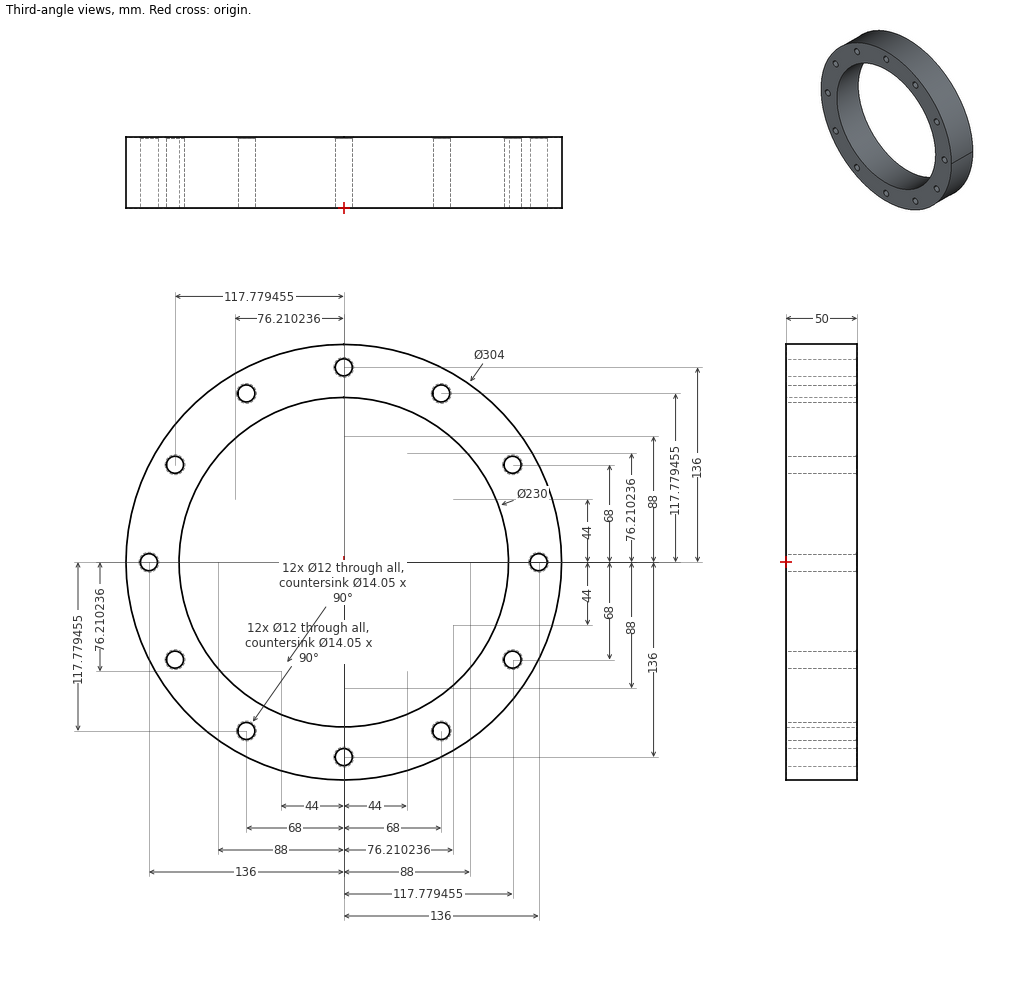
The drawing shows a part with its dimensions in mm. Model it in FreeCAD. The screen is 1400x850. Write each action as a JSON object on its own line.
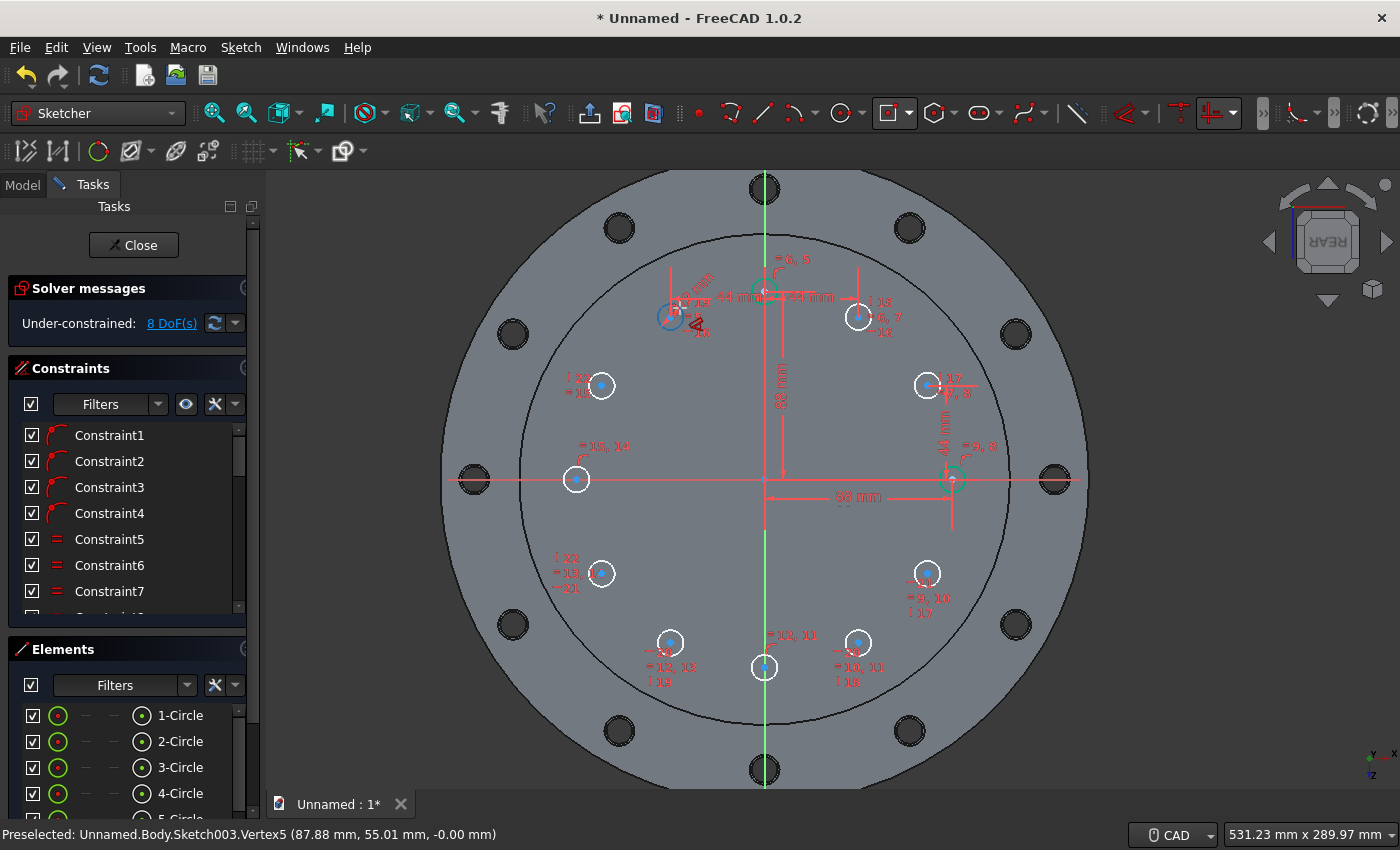
{"action": "left_click", "coordinate": [927, 574]}
{"action": "left_click", "coordinate": [961, 527]}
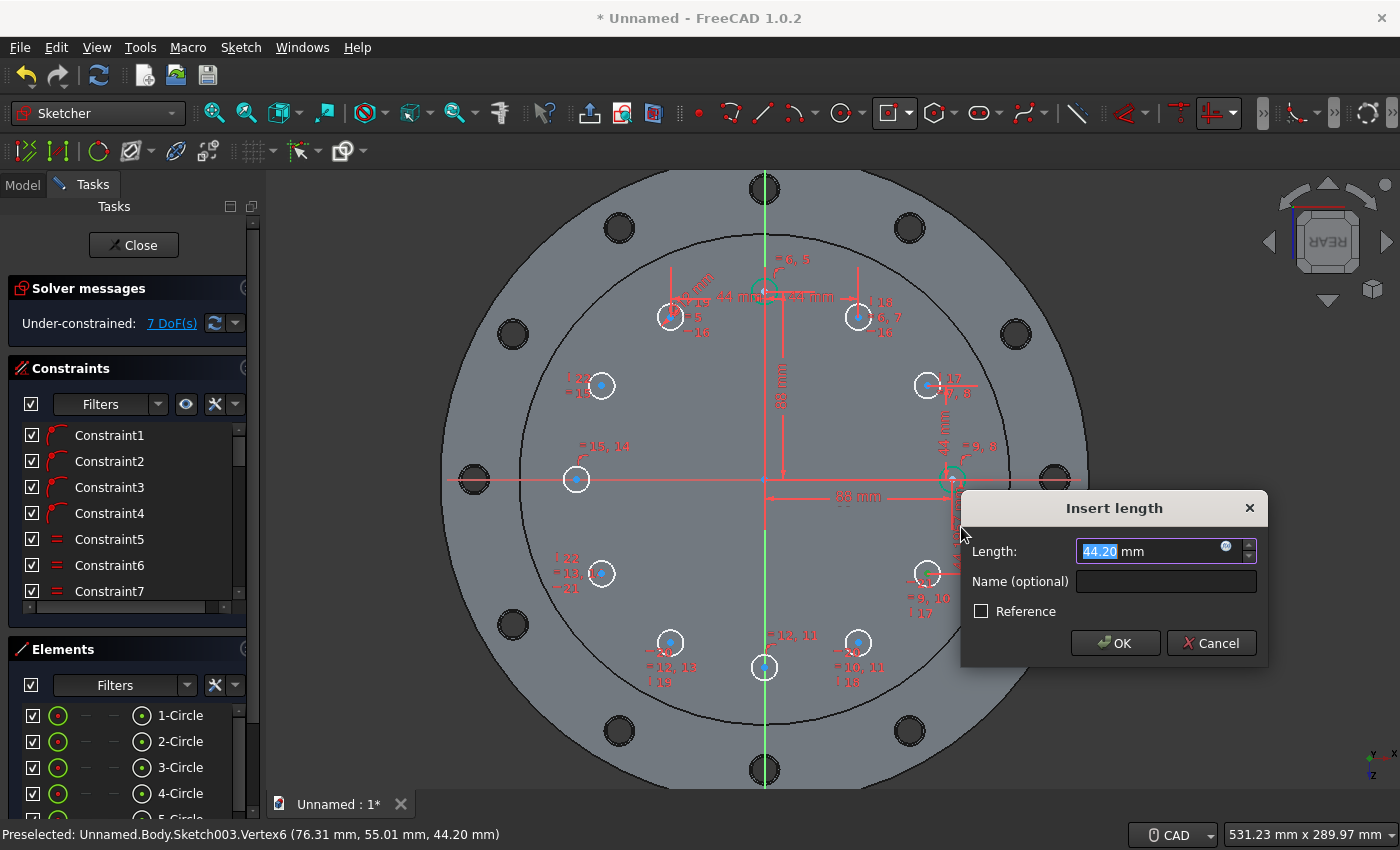
{"action": "type", "text": "44"}
{"action": "key", "text": "Return"}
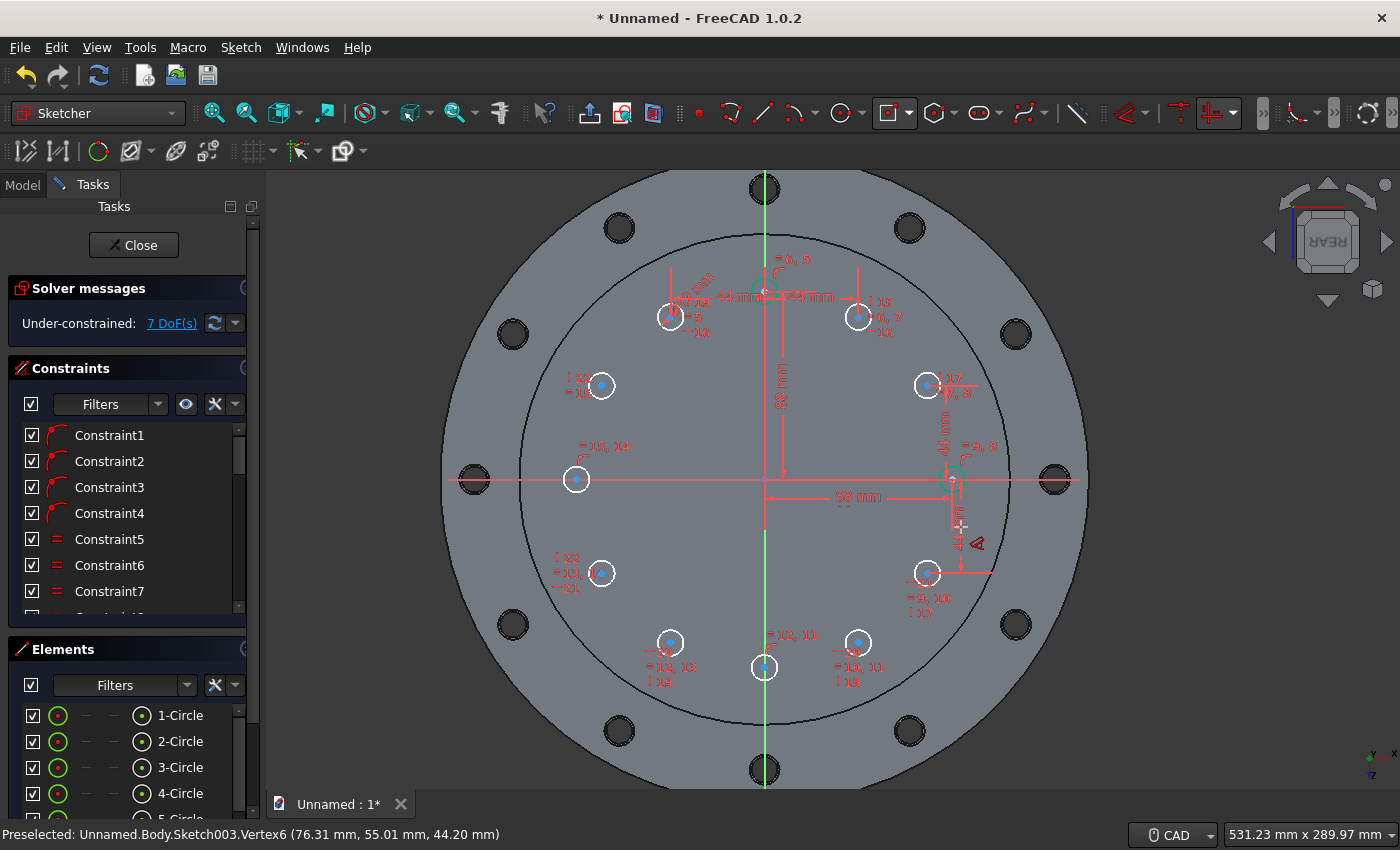
{"action": "left_click", "coordinate": [765, 668]}
{"action": "left_click", "coordinate": [799, 574]}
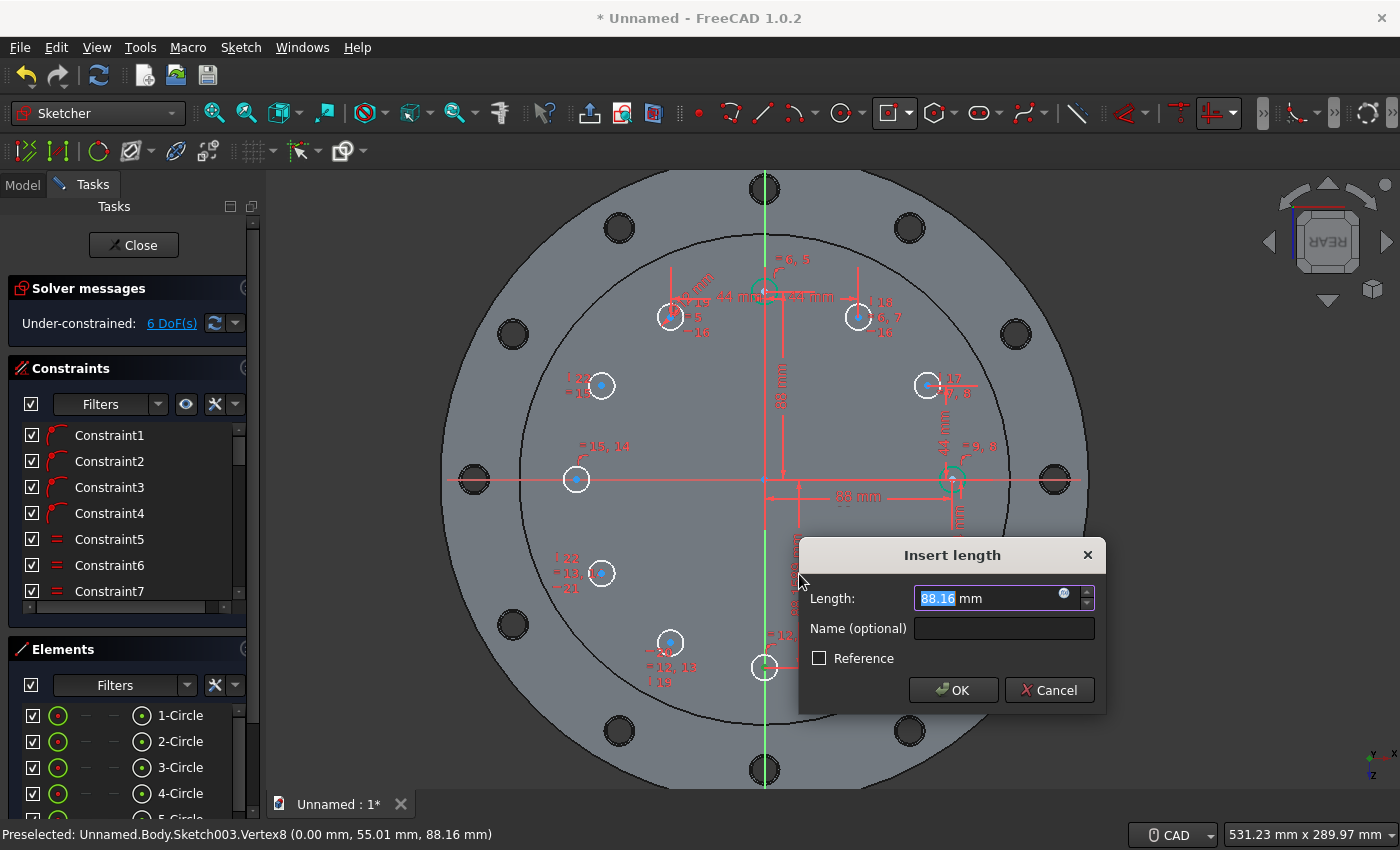
{"action": "type", "text": "88"}
{"action": "key", "text": "Return"}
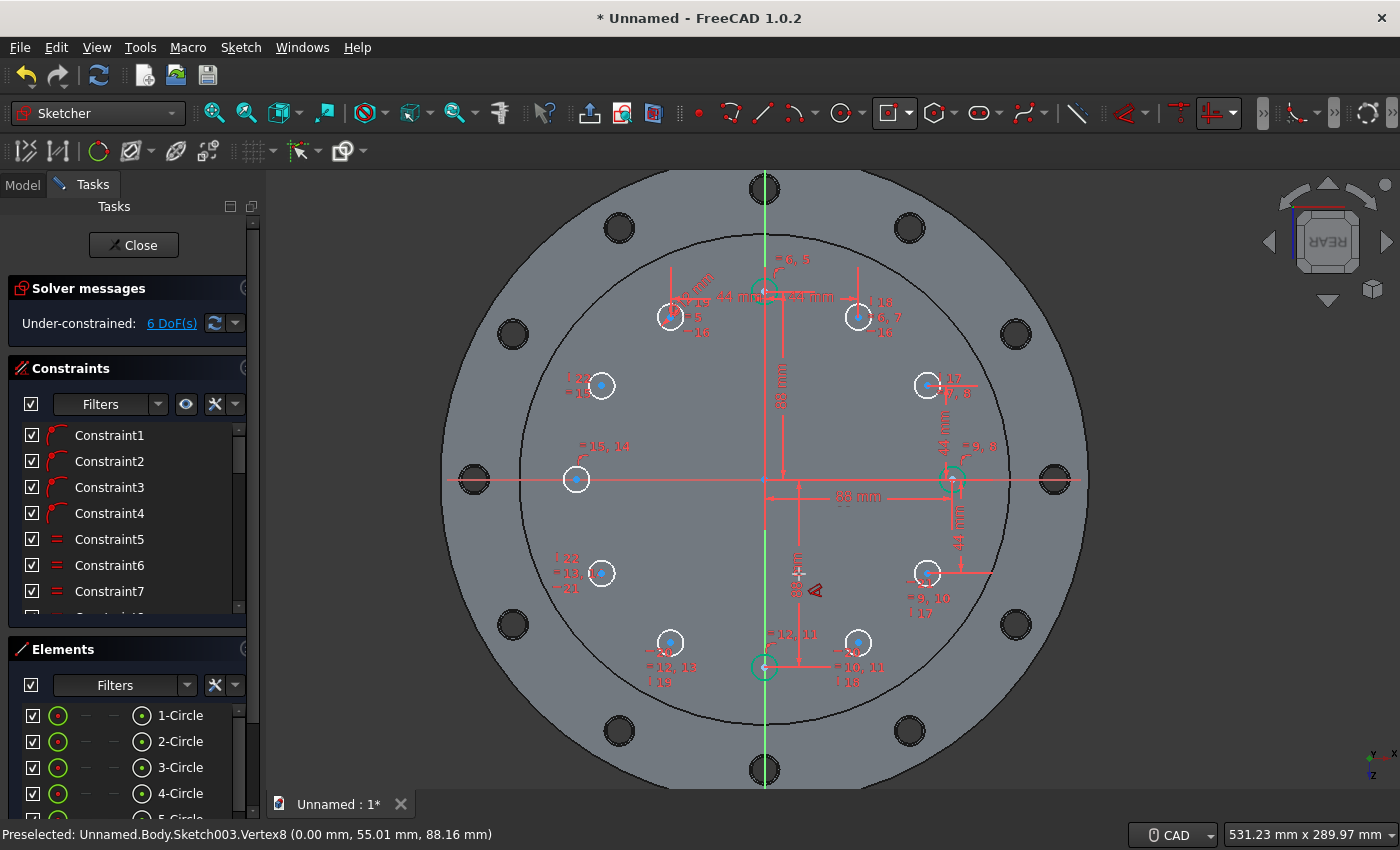
{"action": "left_click", "coordinate": [577, 479]}
{"action": "left_click", "coordinate": [671, 513]}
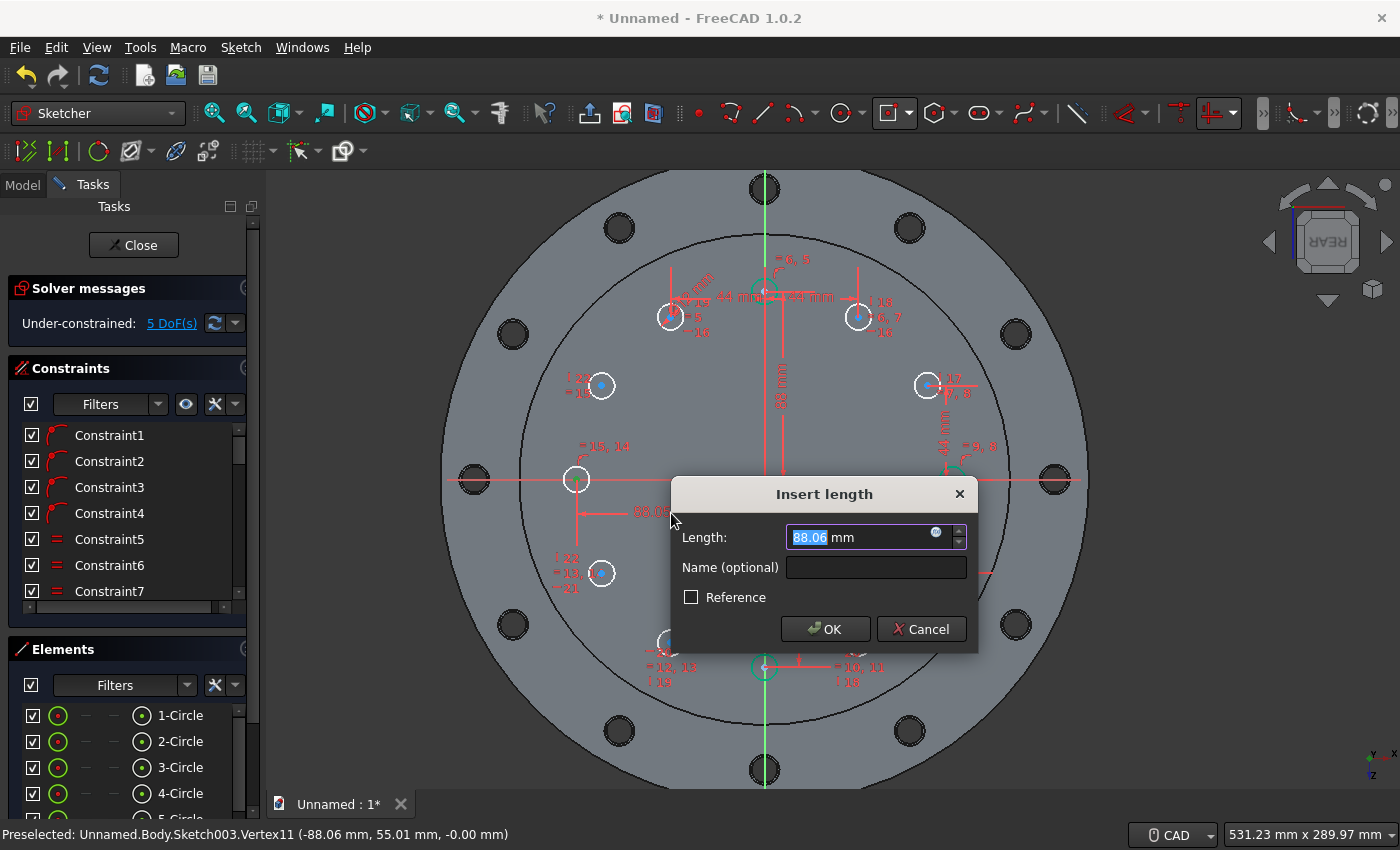
{"action": "type", "text": "88"}
{"action": "key", "text": "Return"}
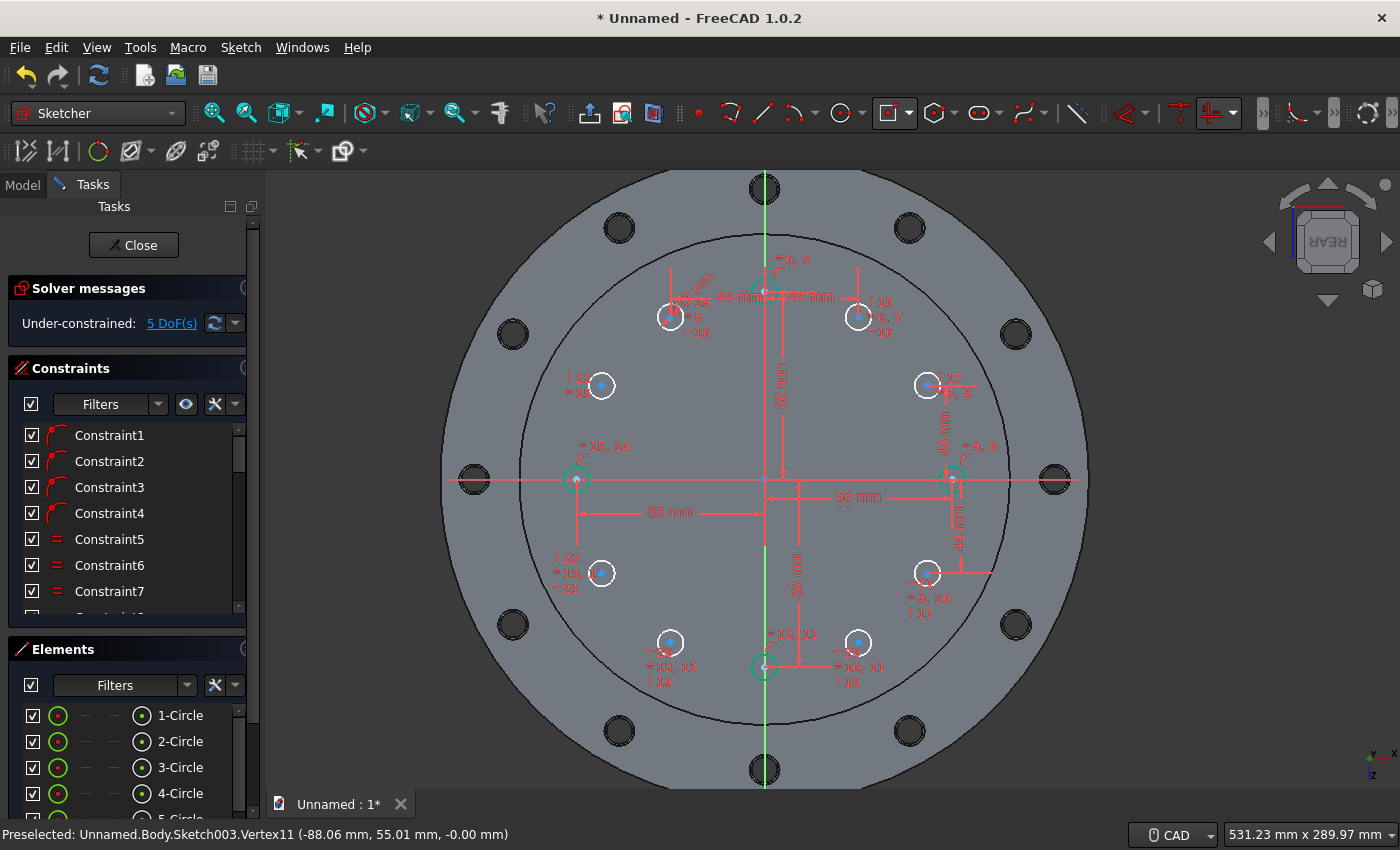
{"action": "left_click", "coordinate": [602, 386]}
{"action": "left_click", "coordinate": [568, 433]}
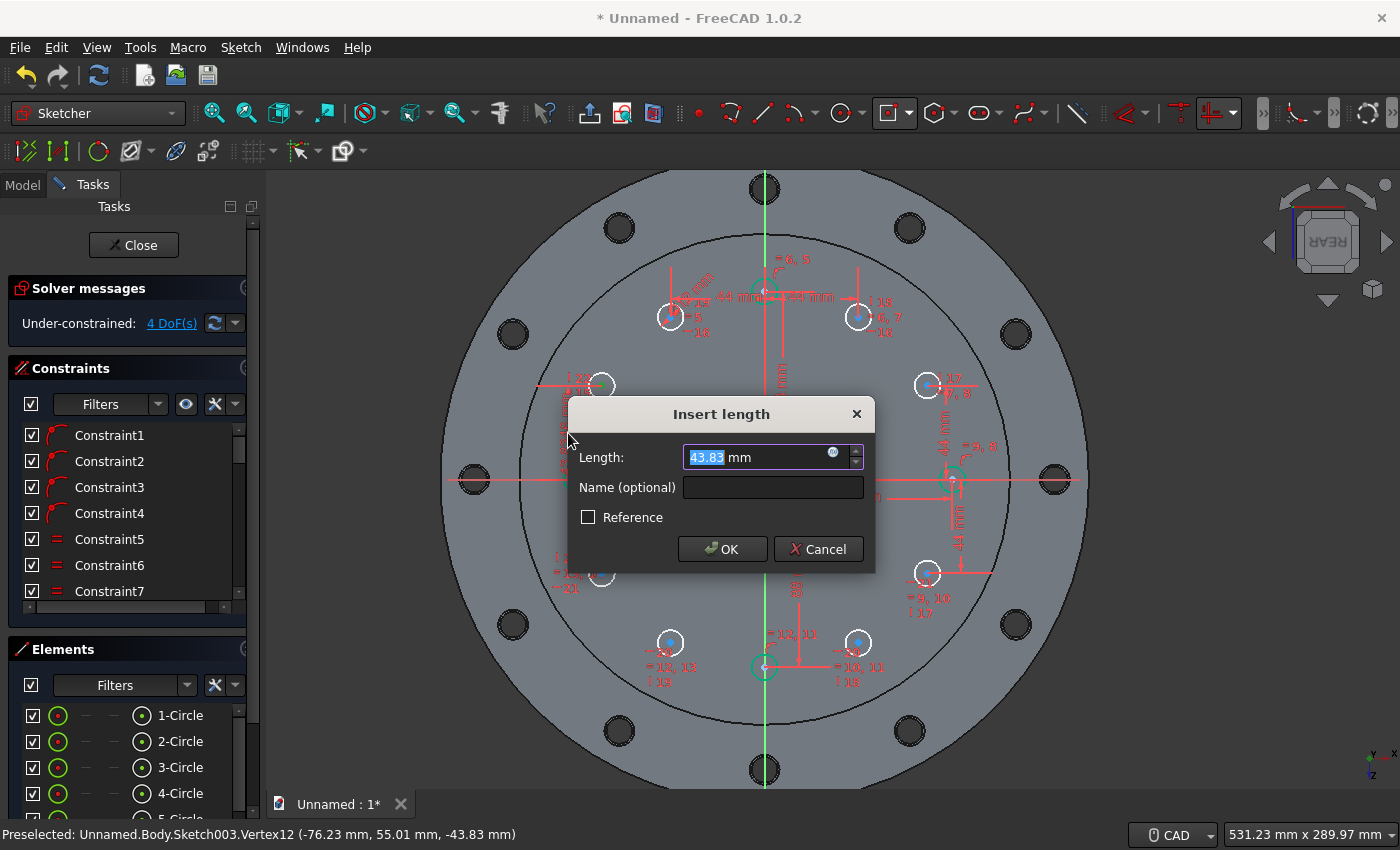
{"action": "type", "text": "44"}
{"action": "key", "text": "Return"}